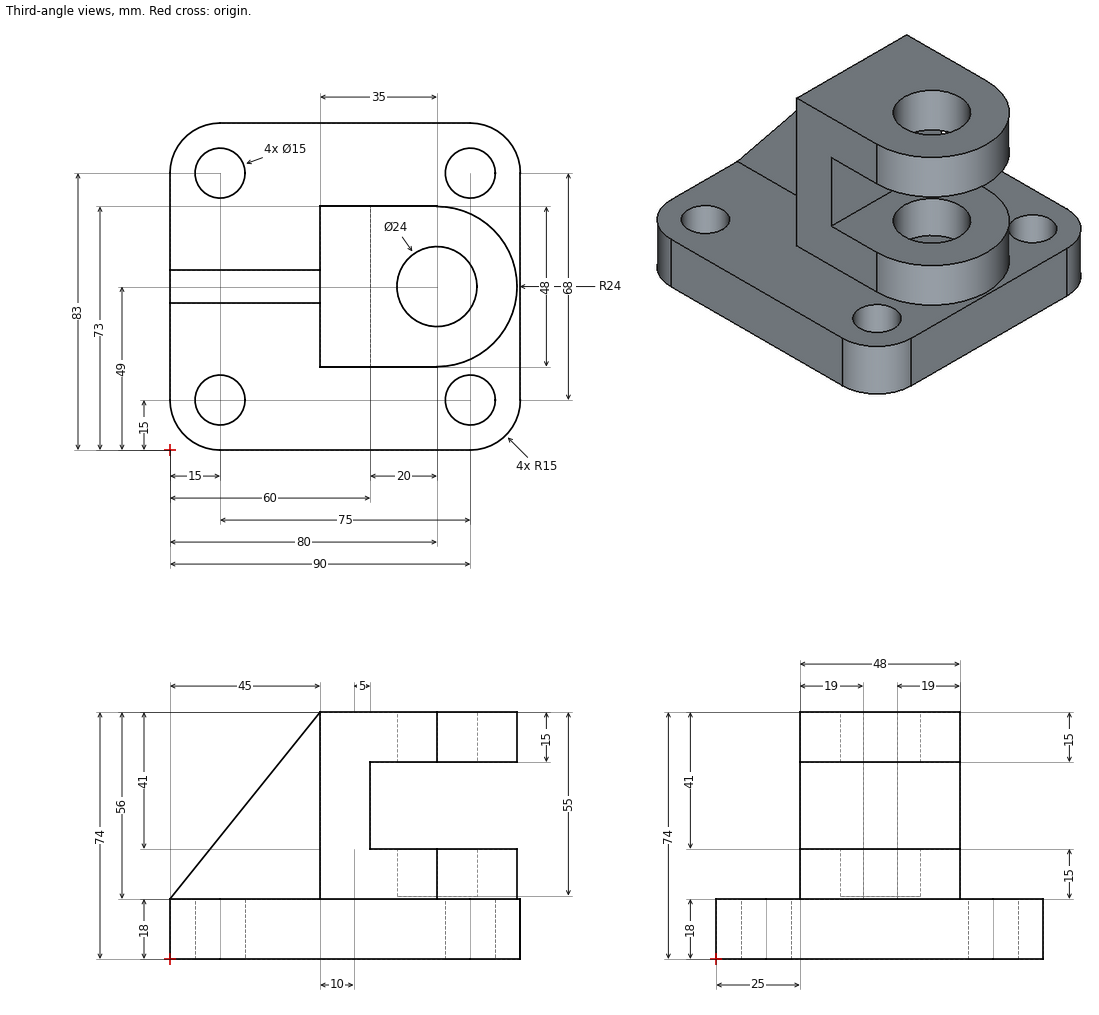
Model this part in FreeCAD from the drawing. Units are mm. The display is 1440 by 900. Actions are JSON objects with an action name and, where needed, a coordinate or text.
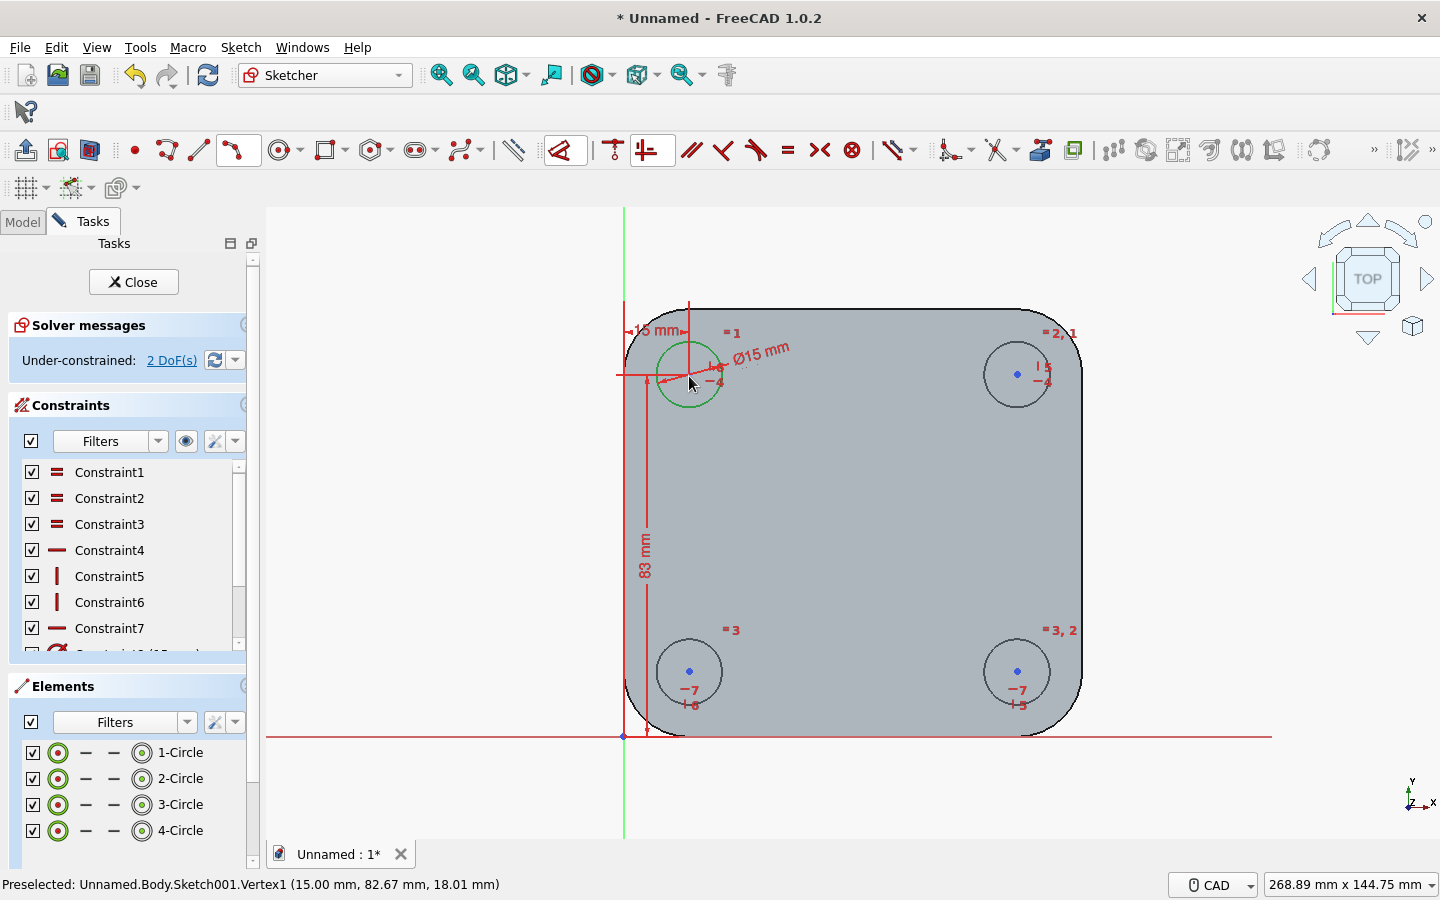
{"action": "left_click", "coordinate": [1017, 375]}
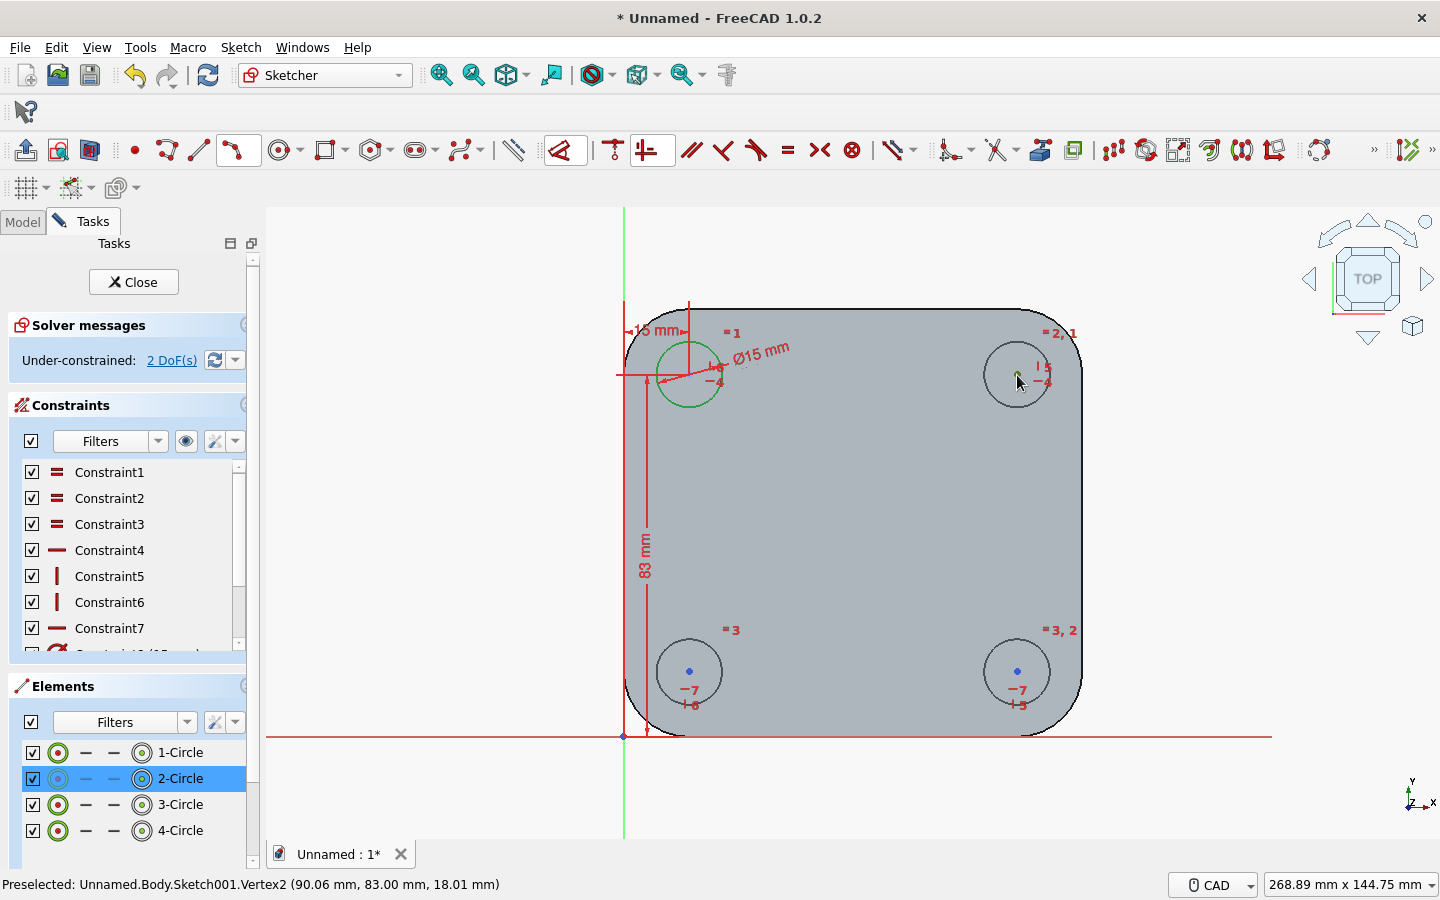
{"action": "left_click", "coordinate": [582, 150]}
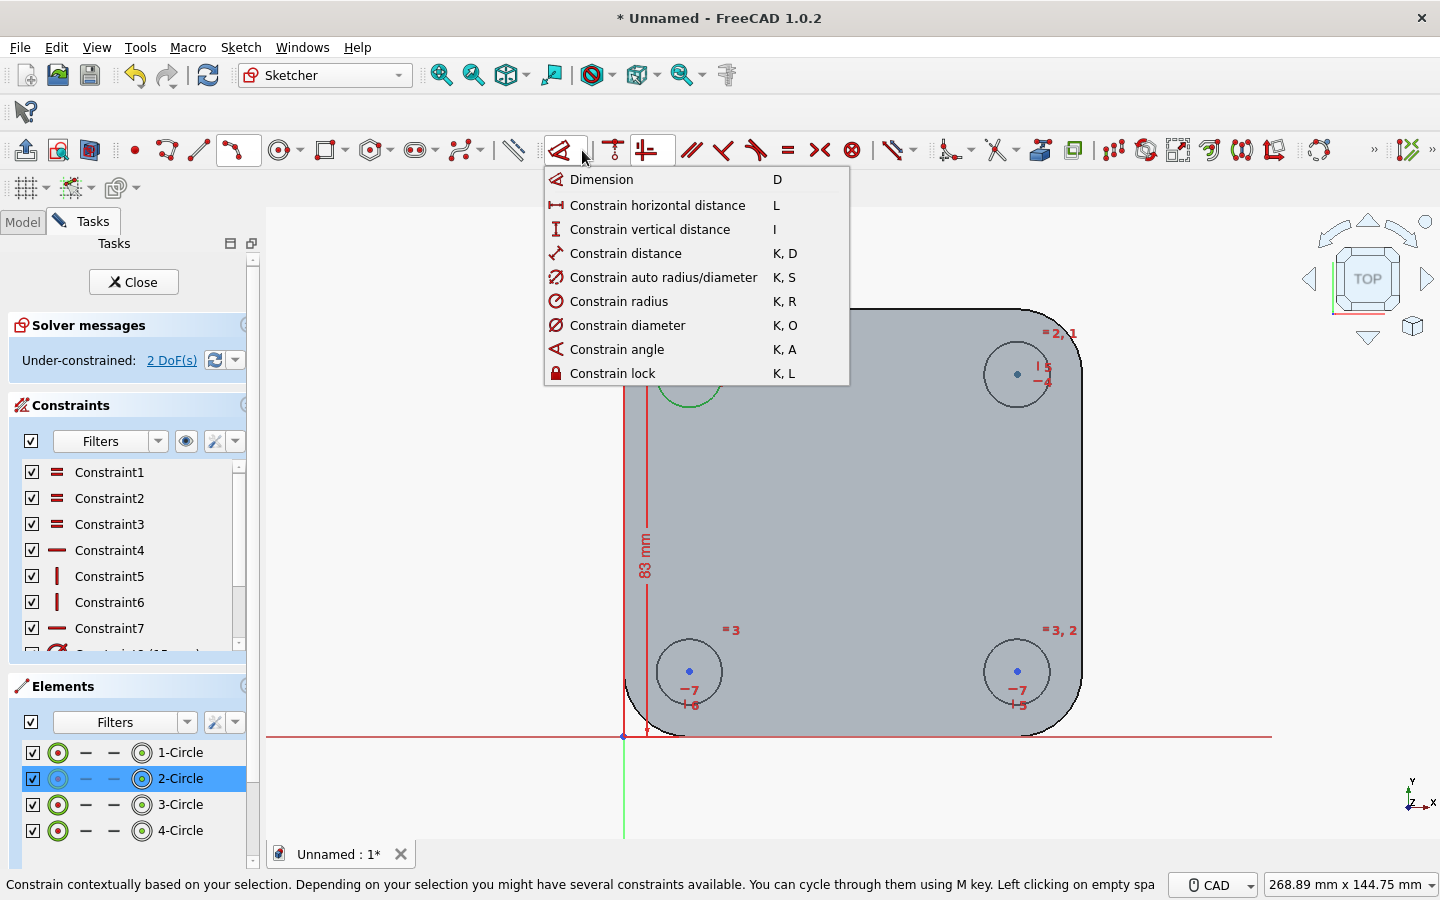
{"action": "left_click", "coordinate": [697, 205]}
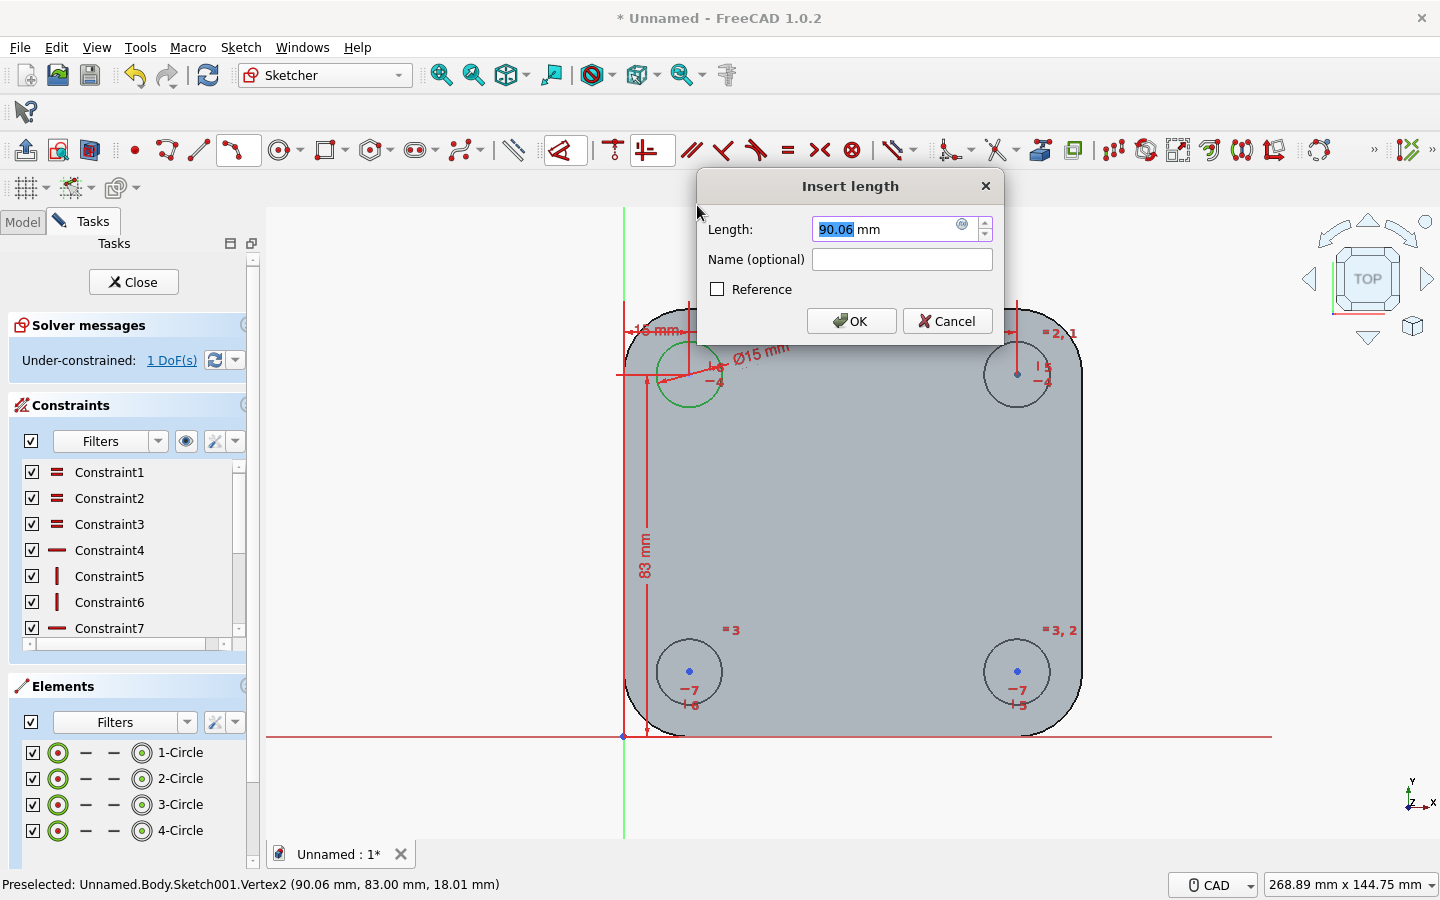
{"action": "type", "text": "90"}
{"action": "key", "text": "Return"}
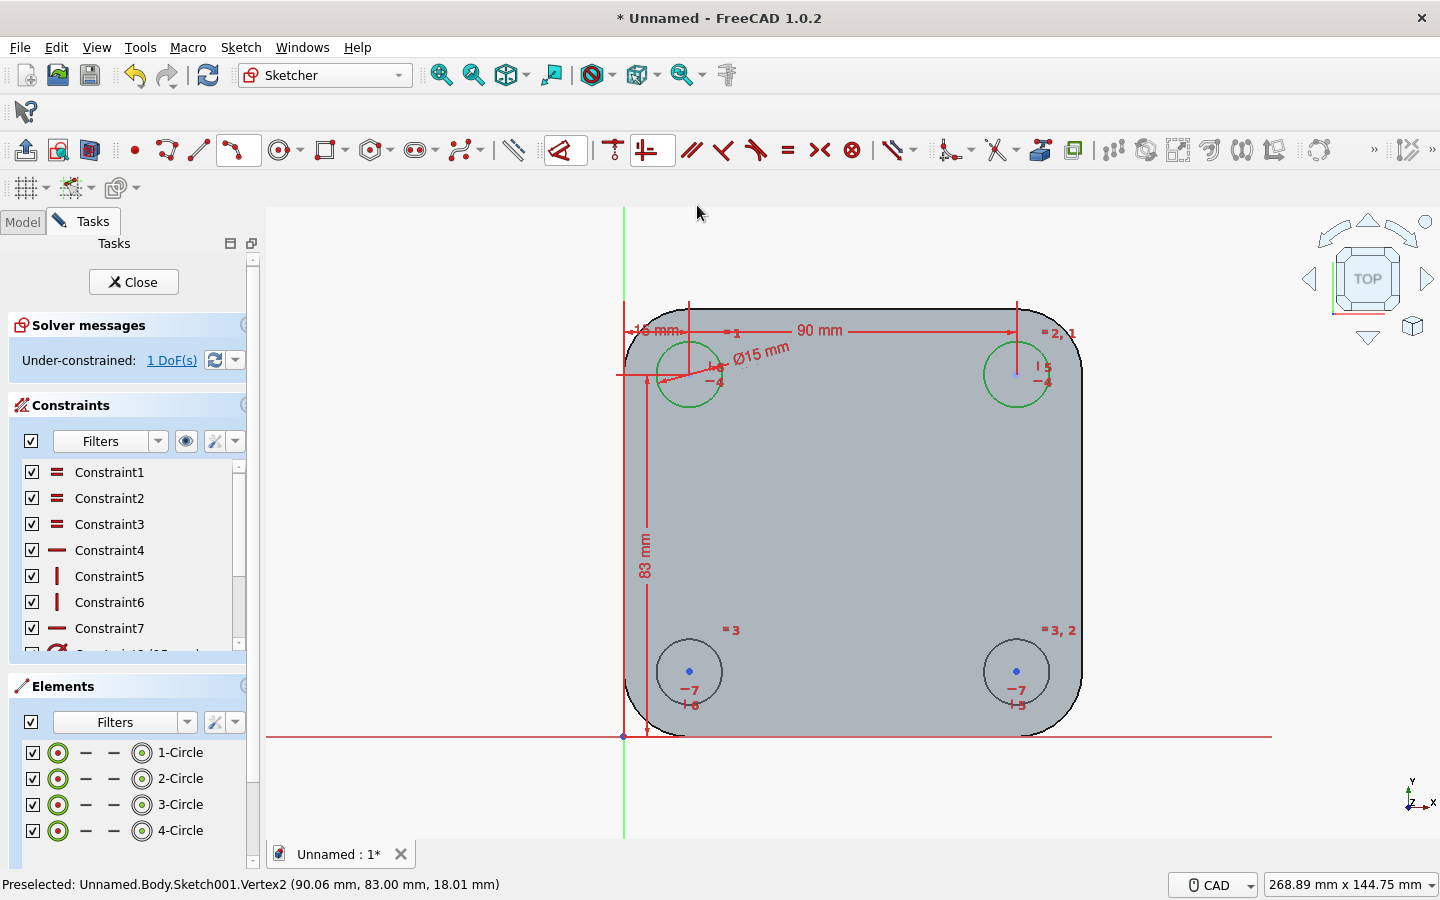
{"action": "left_click", "coordinate": [1017, 672]}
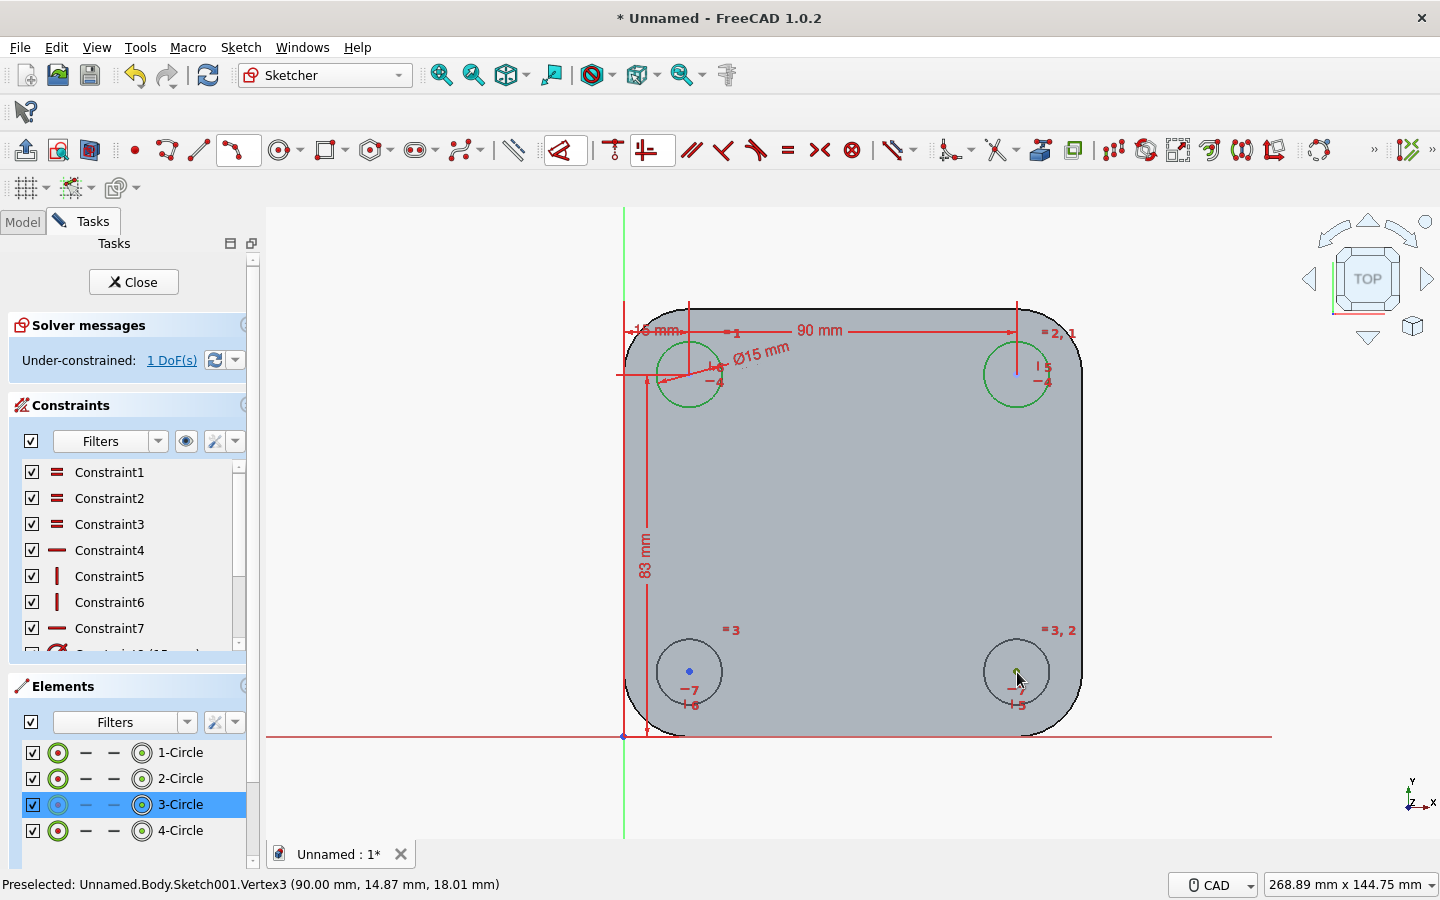
{"action": "left_click", "coordinate": [582, 150]}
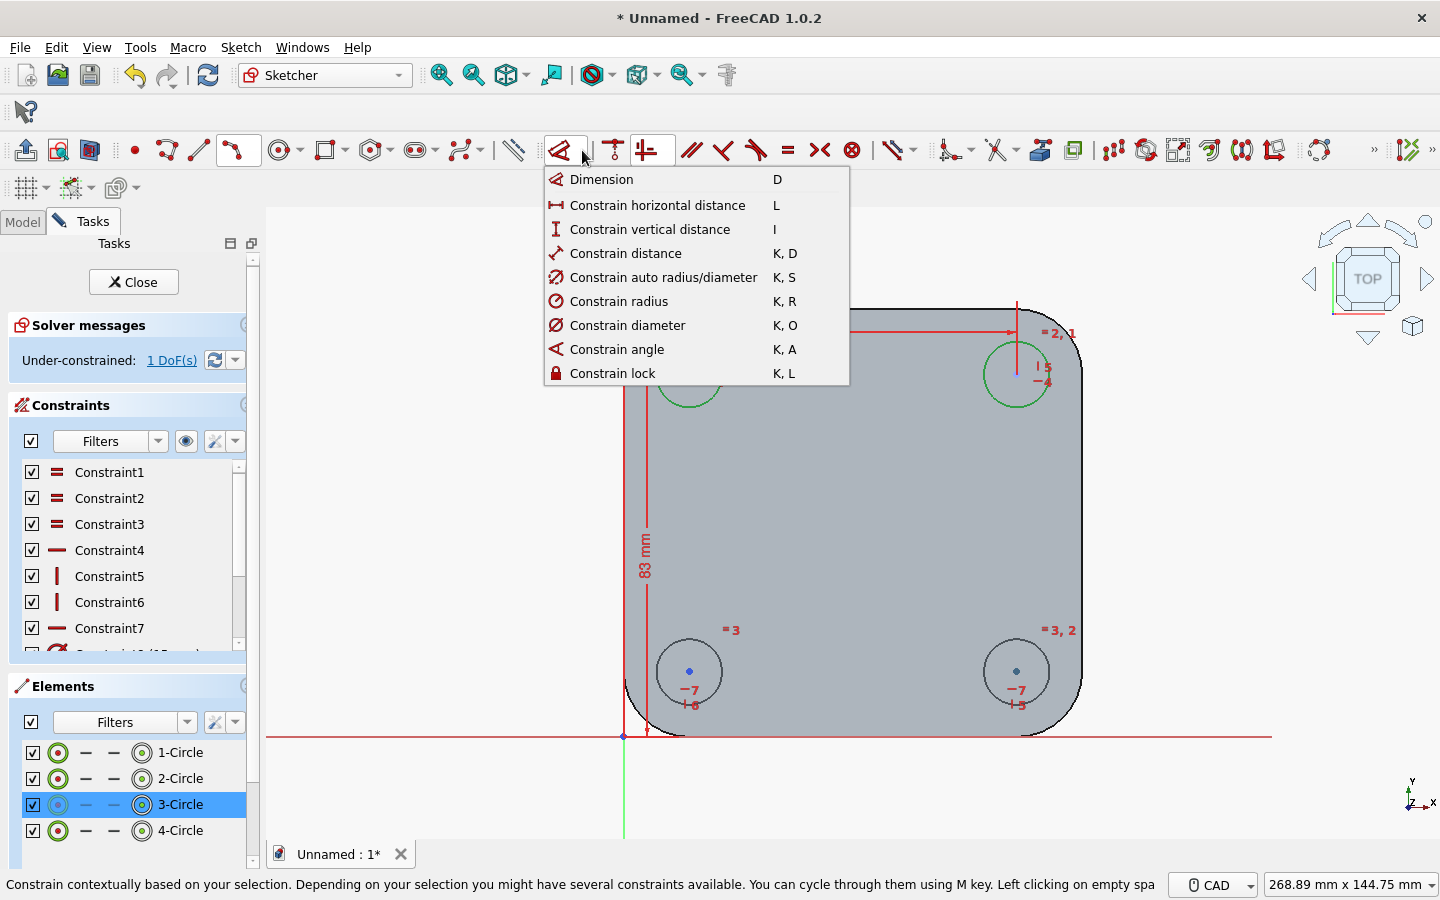
{"action": "left_click", "coordinate": [697, 229]}